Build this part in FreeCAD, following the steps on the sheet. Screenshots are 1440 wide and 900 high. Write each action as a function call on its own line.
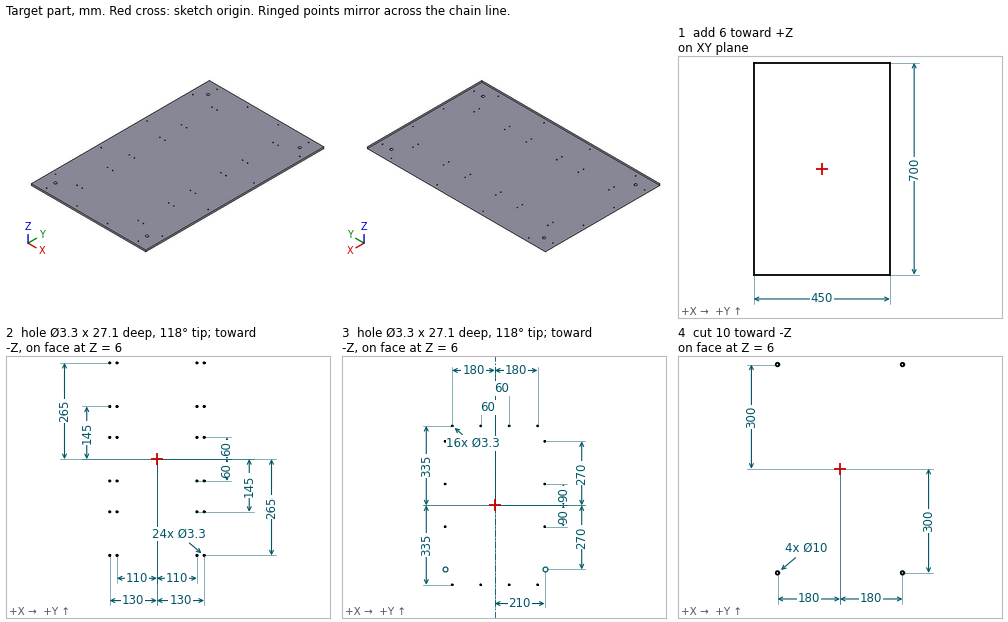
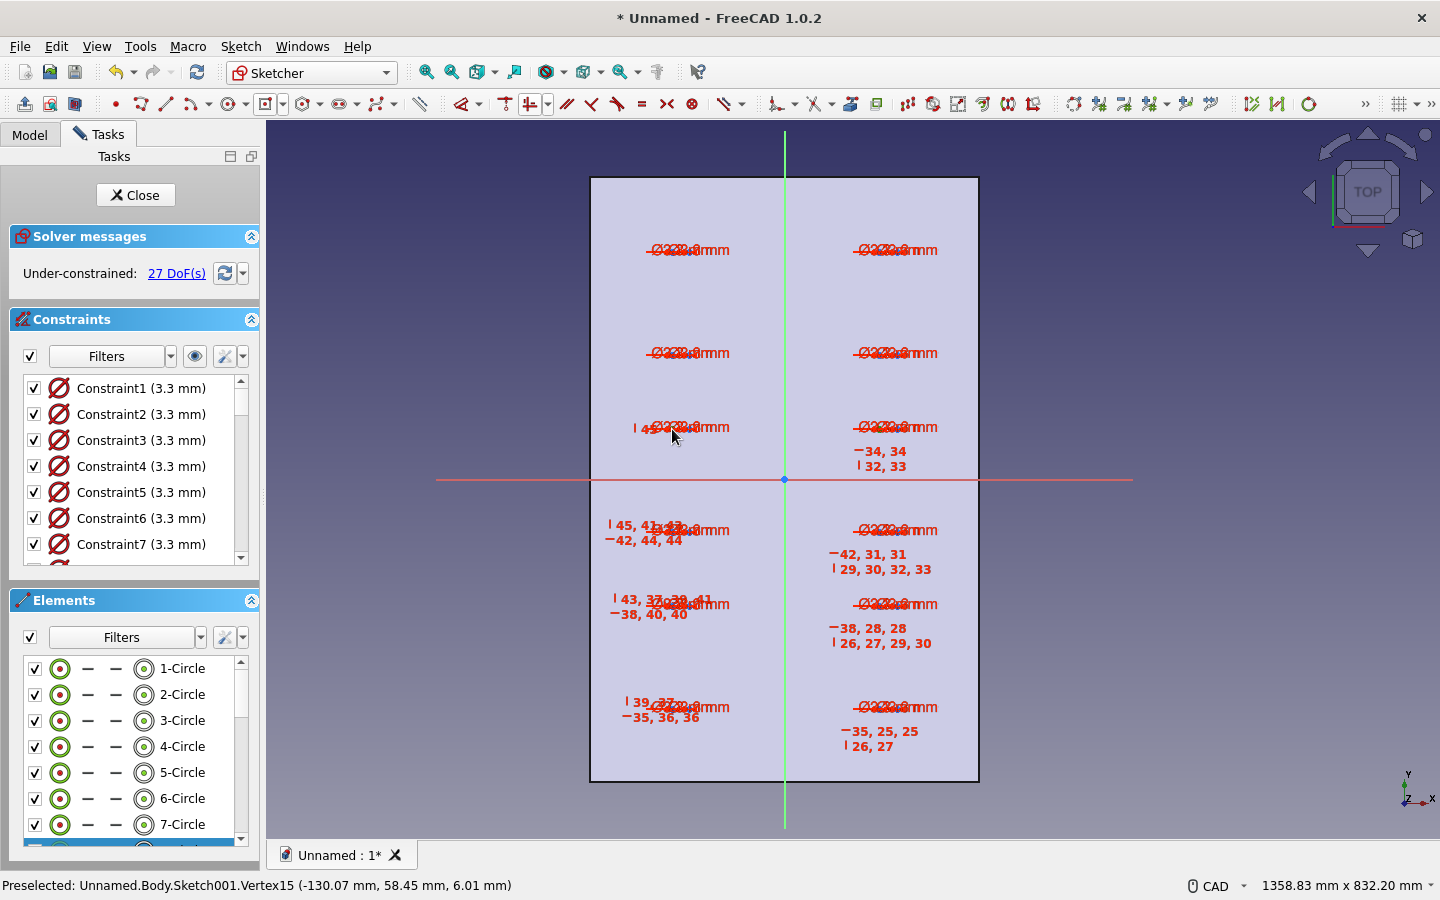
click(548, 104)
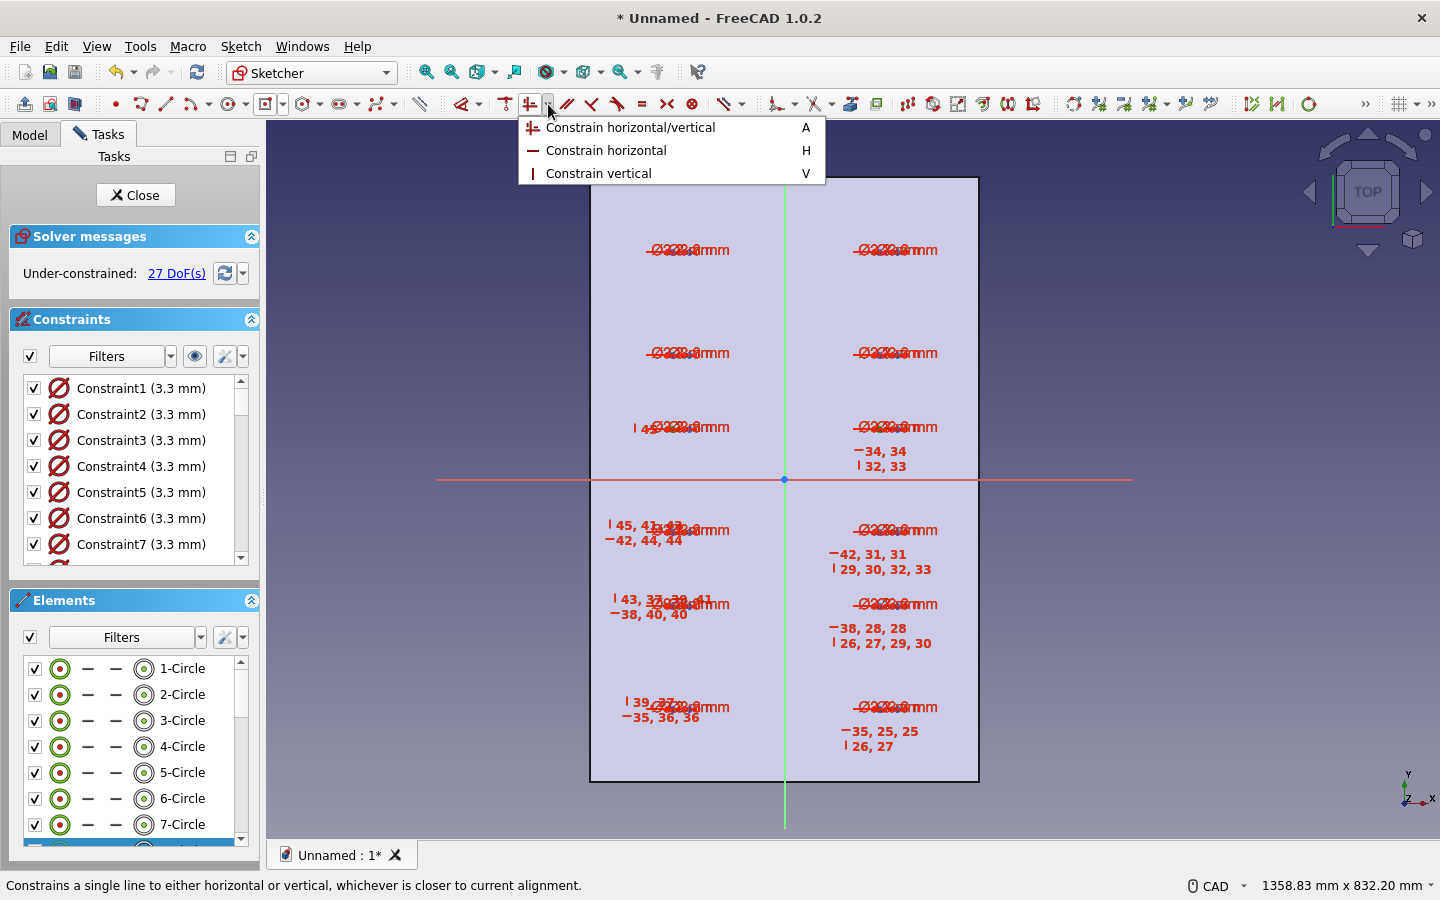
click(672, 150)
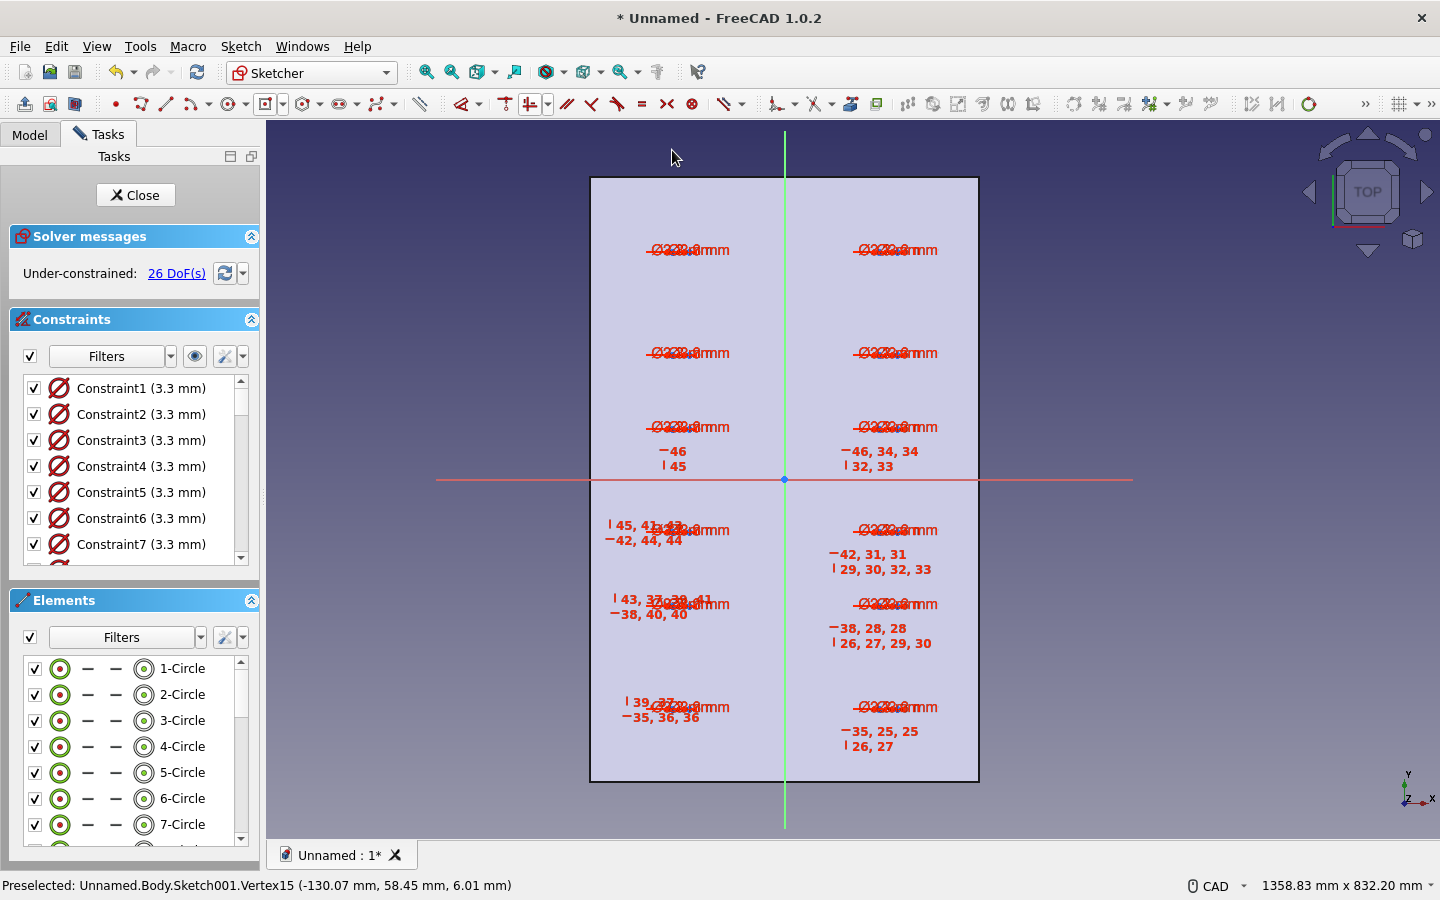
click(689, 532)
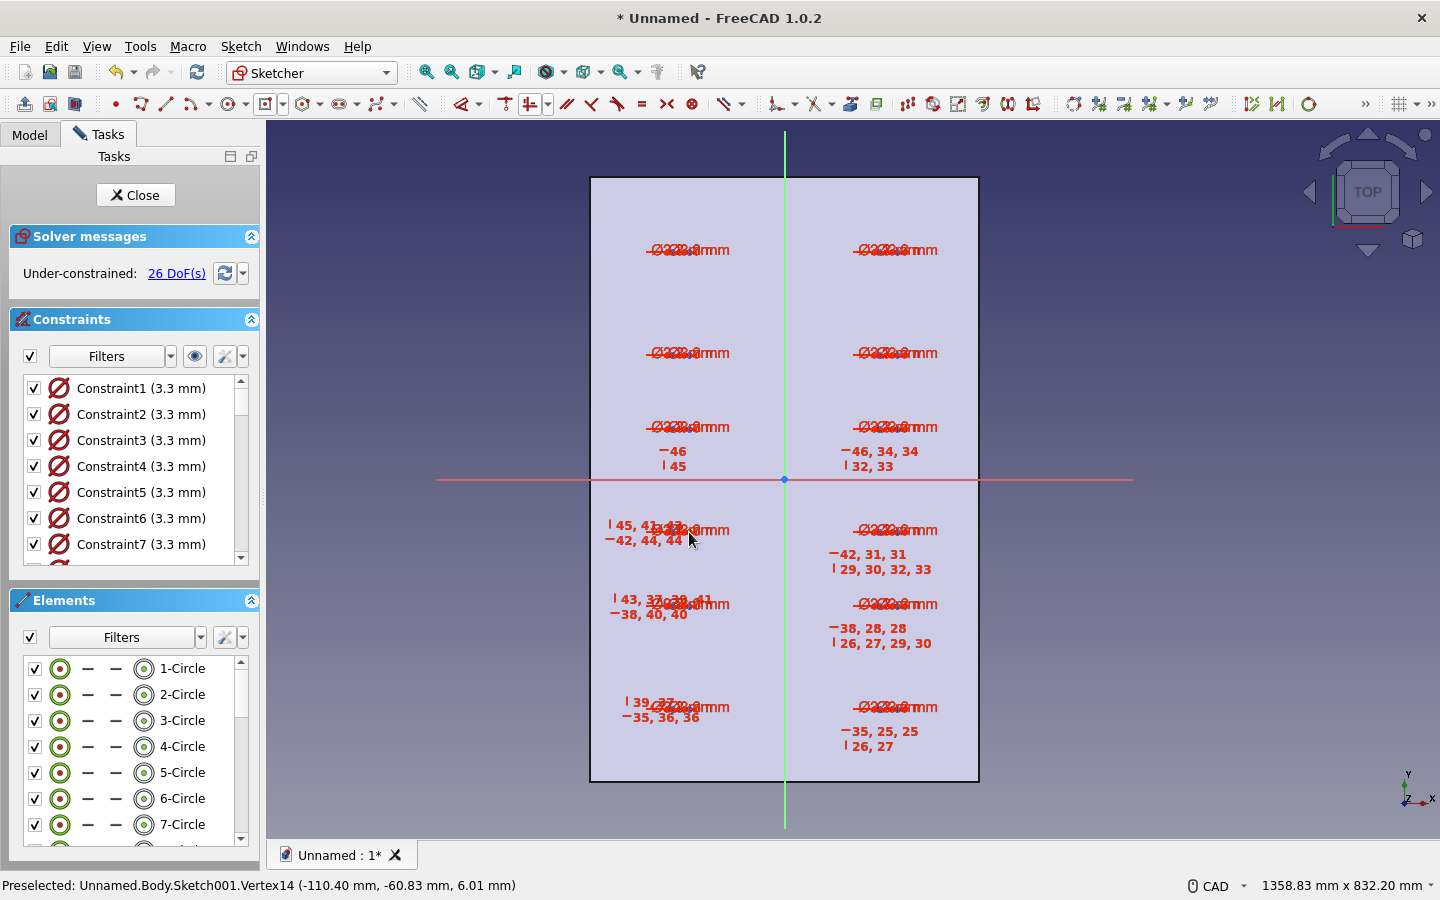
click(689, 429)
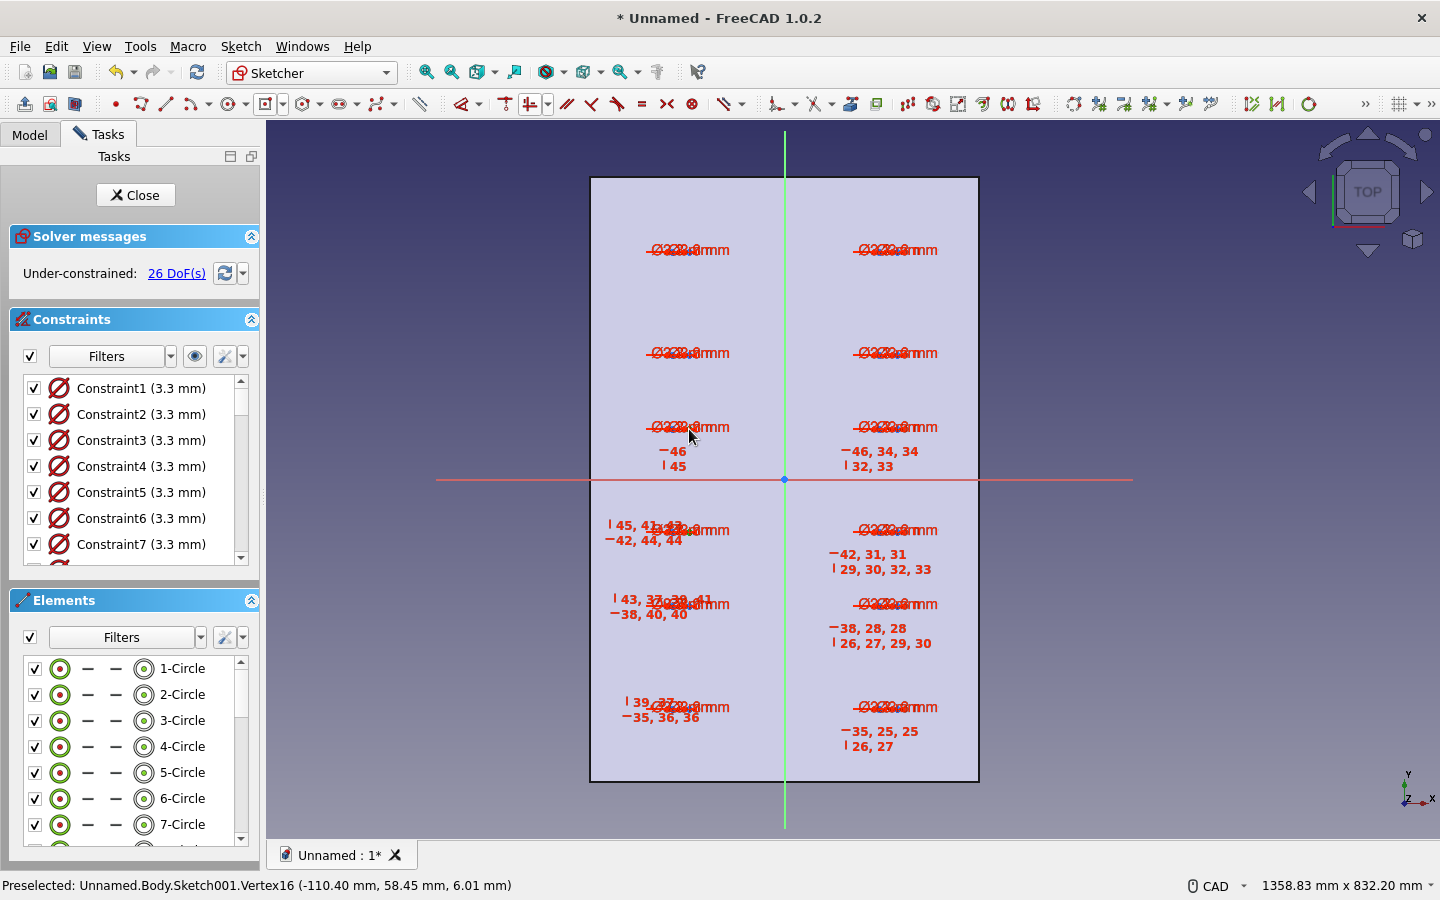
click(548, 104)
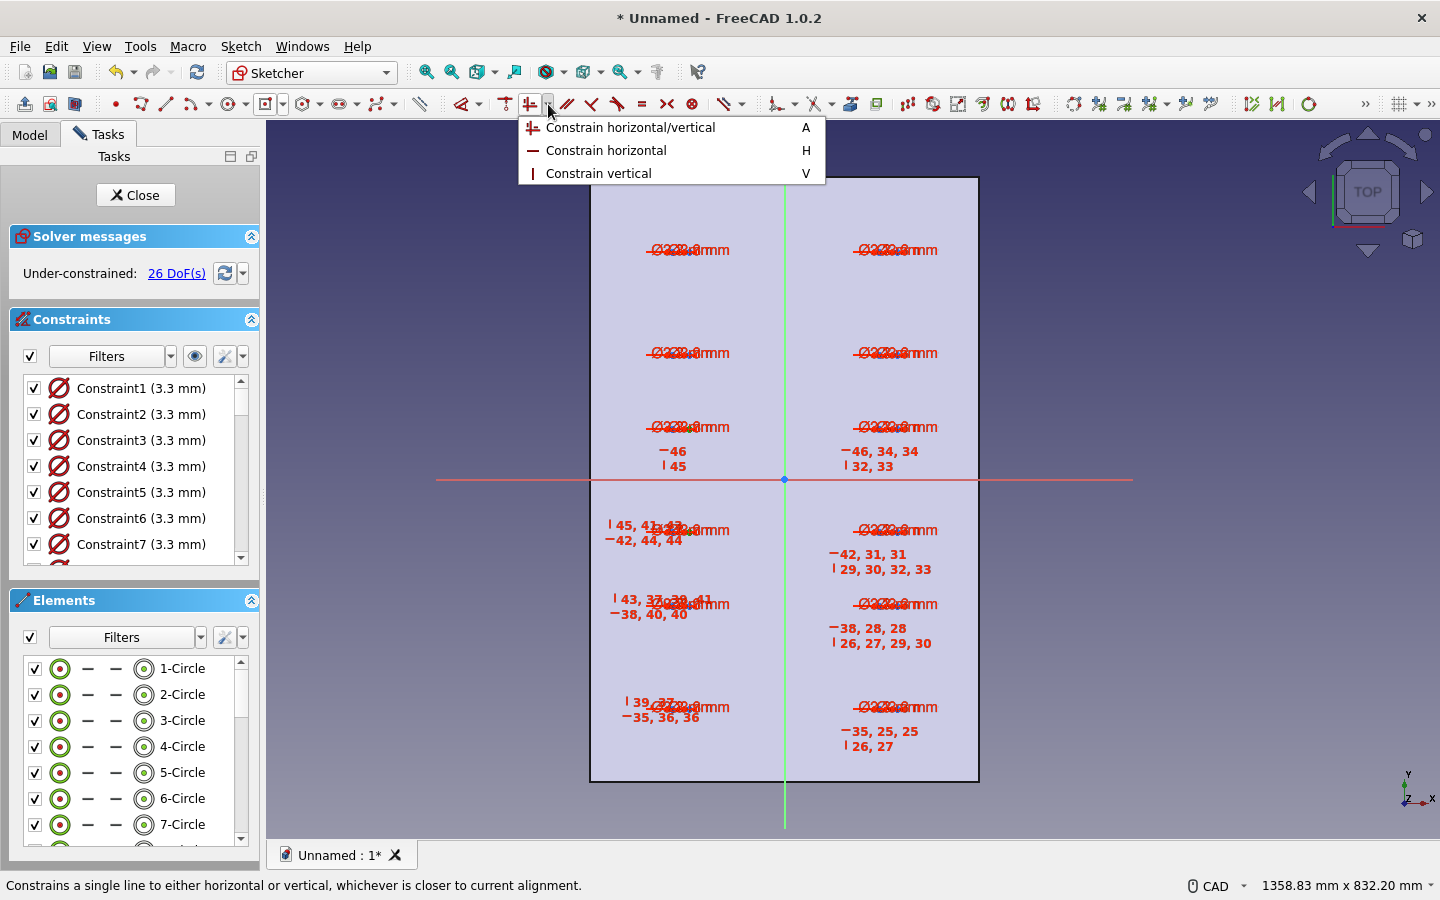
click(672, 174)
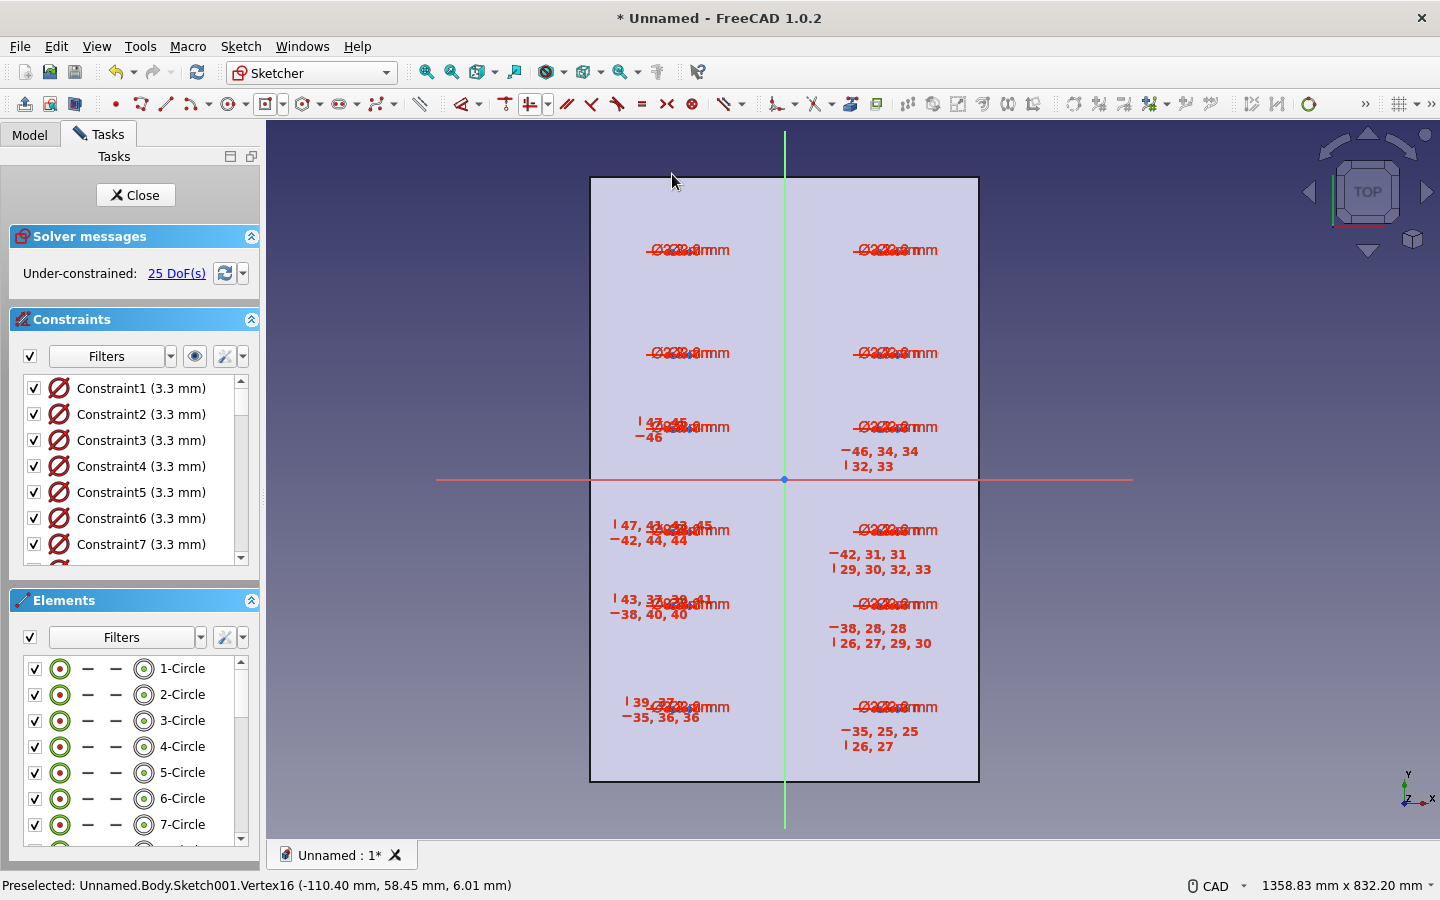
scroll(672, 429, up, 4)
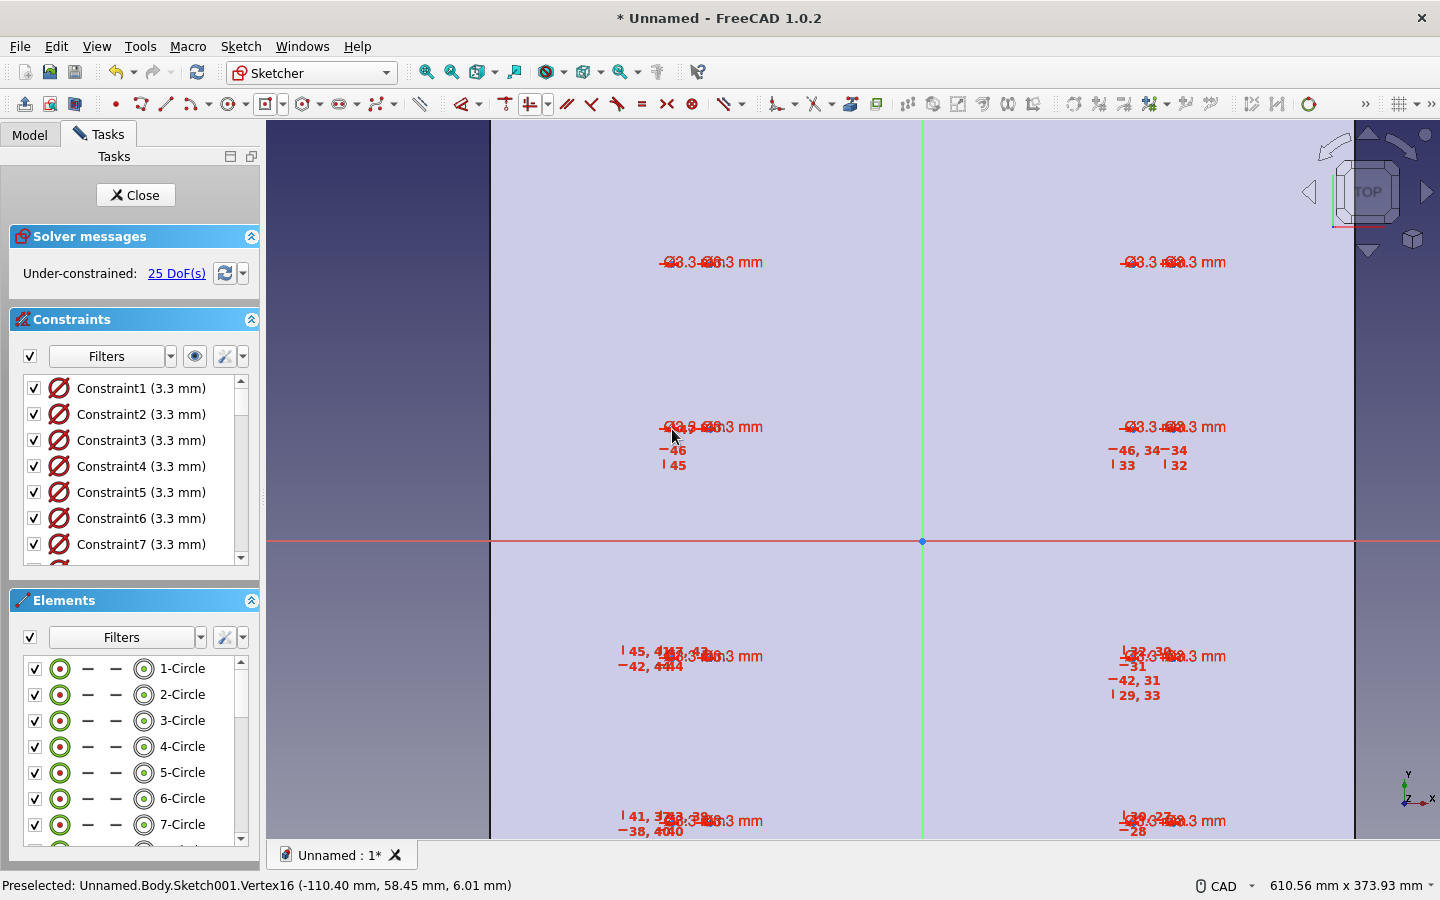
scroll(672, 429, up, 4)